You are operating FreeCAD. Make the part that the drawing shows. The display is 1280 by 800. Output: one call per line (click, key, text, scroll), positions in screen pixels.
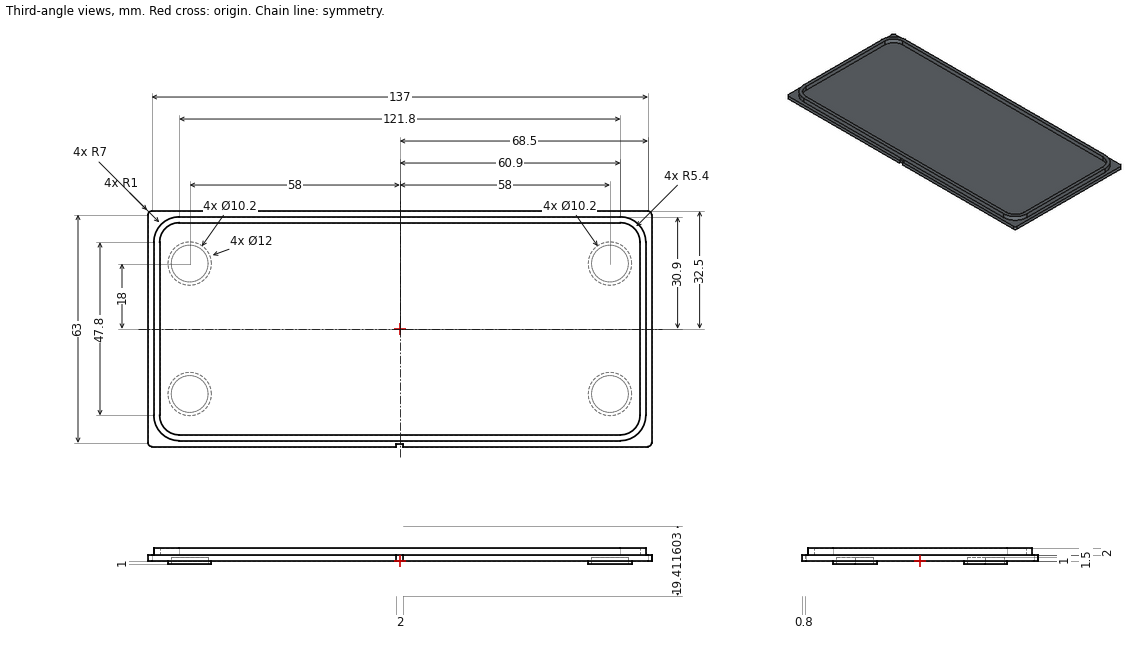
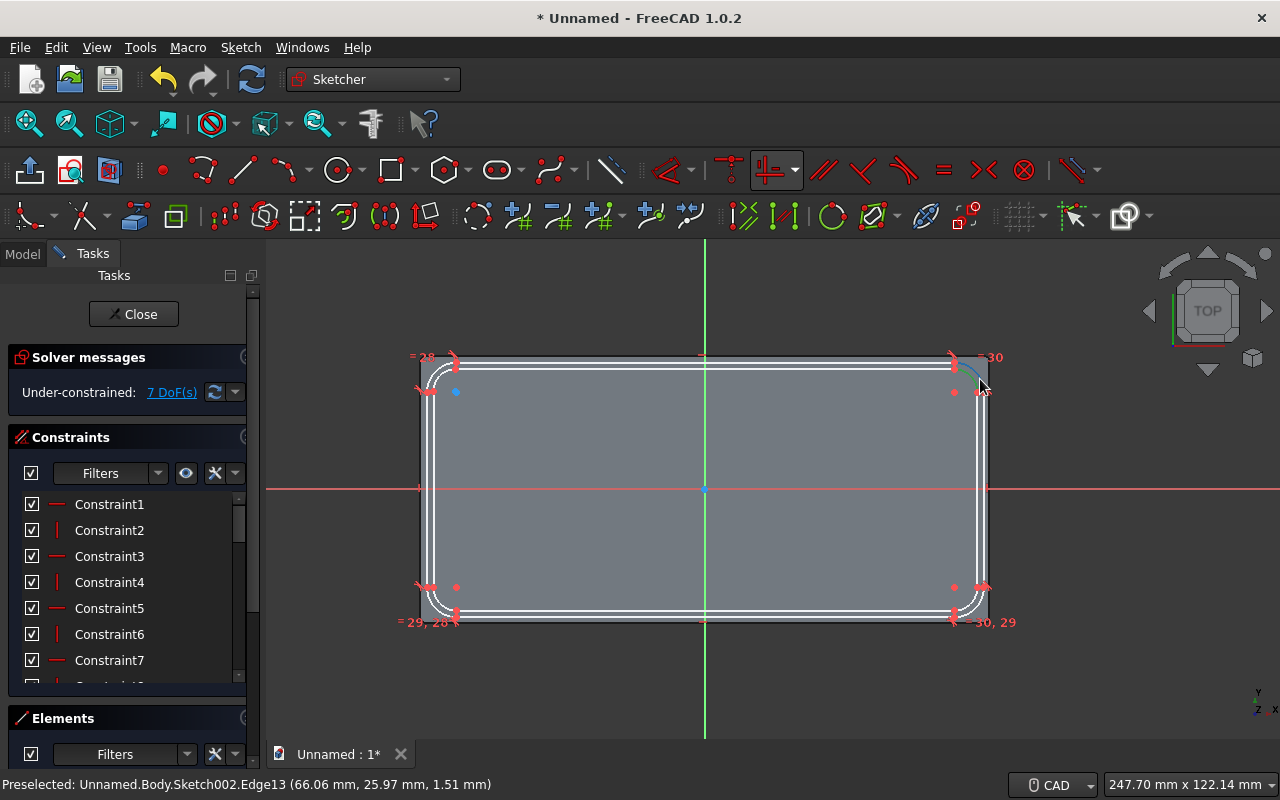
scroll(446, 372, up, 5)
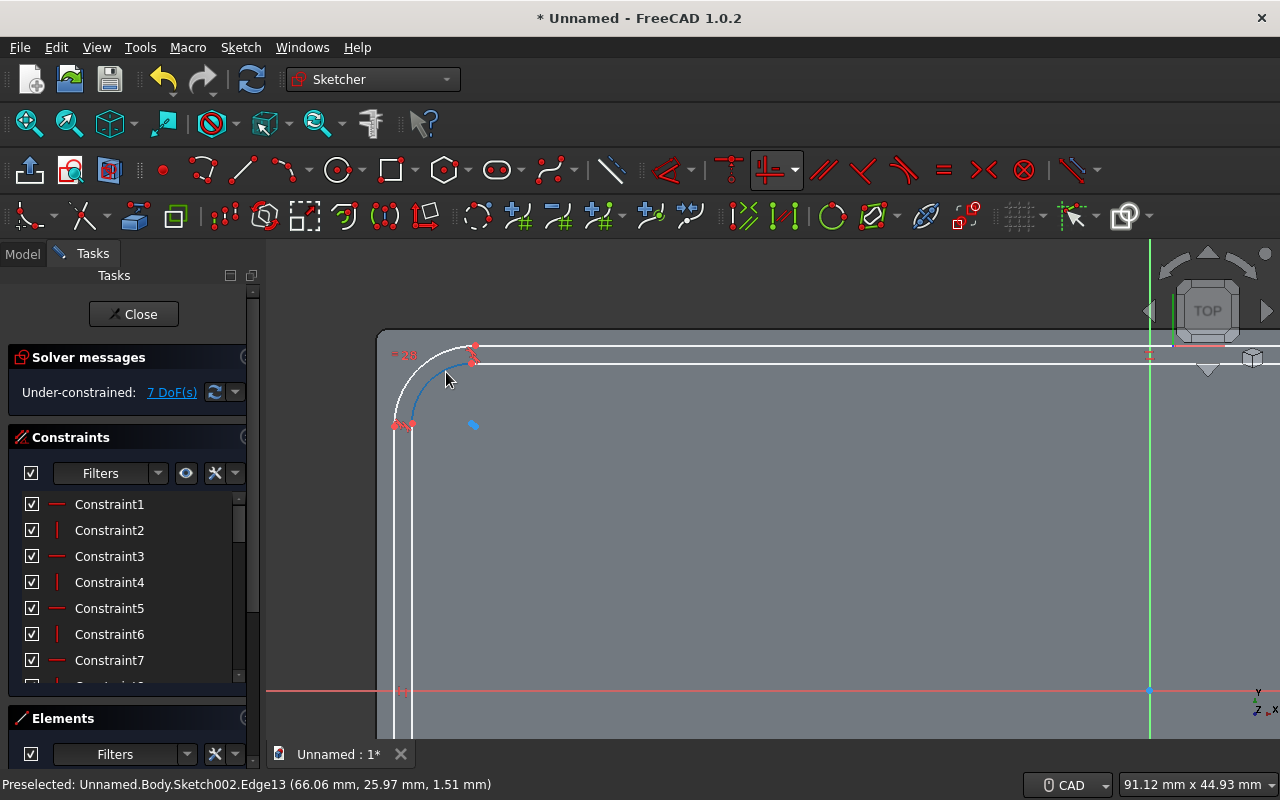
click(445, 370)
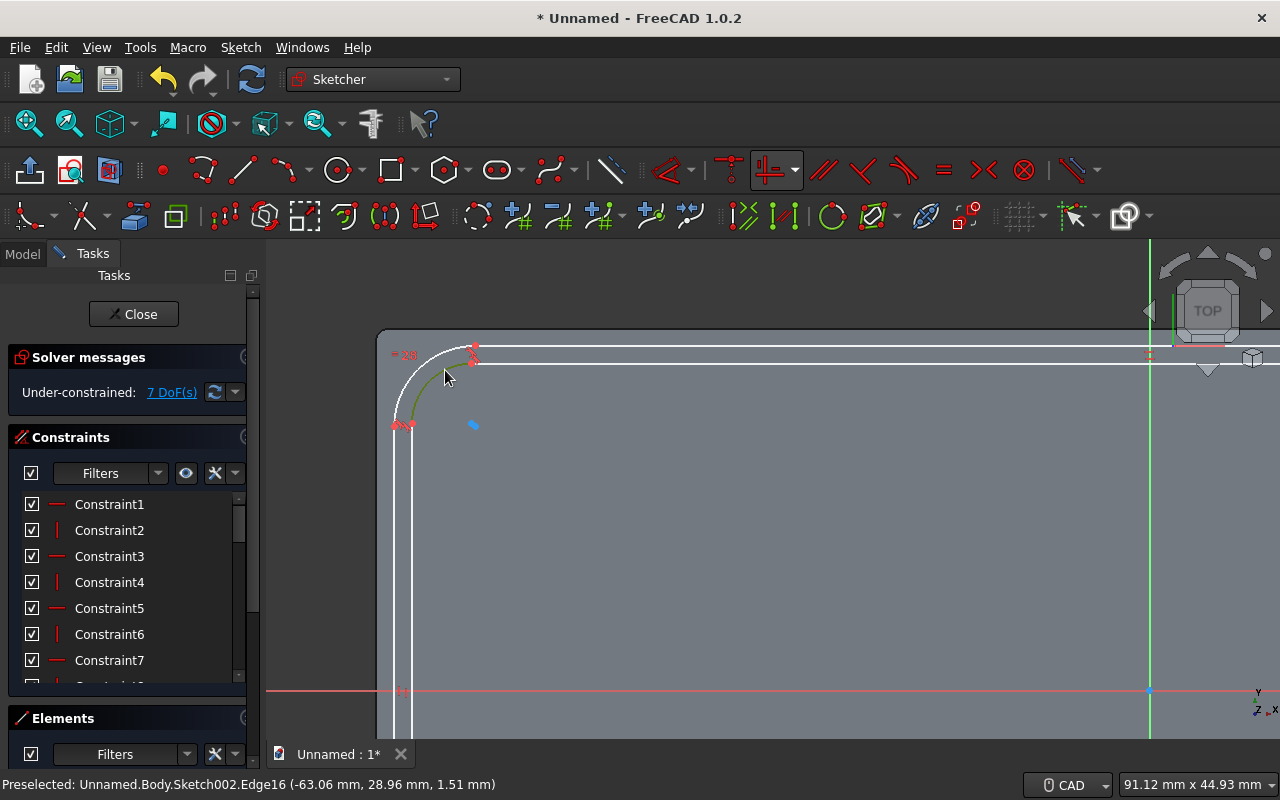
click(944, 170)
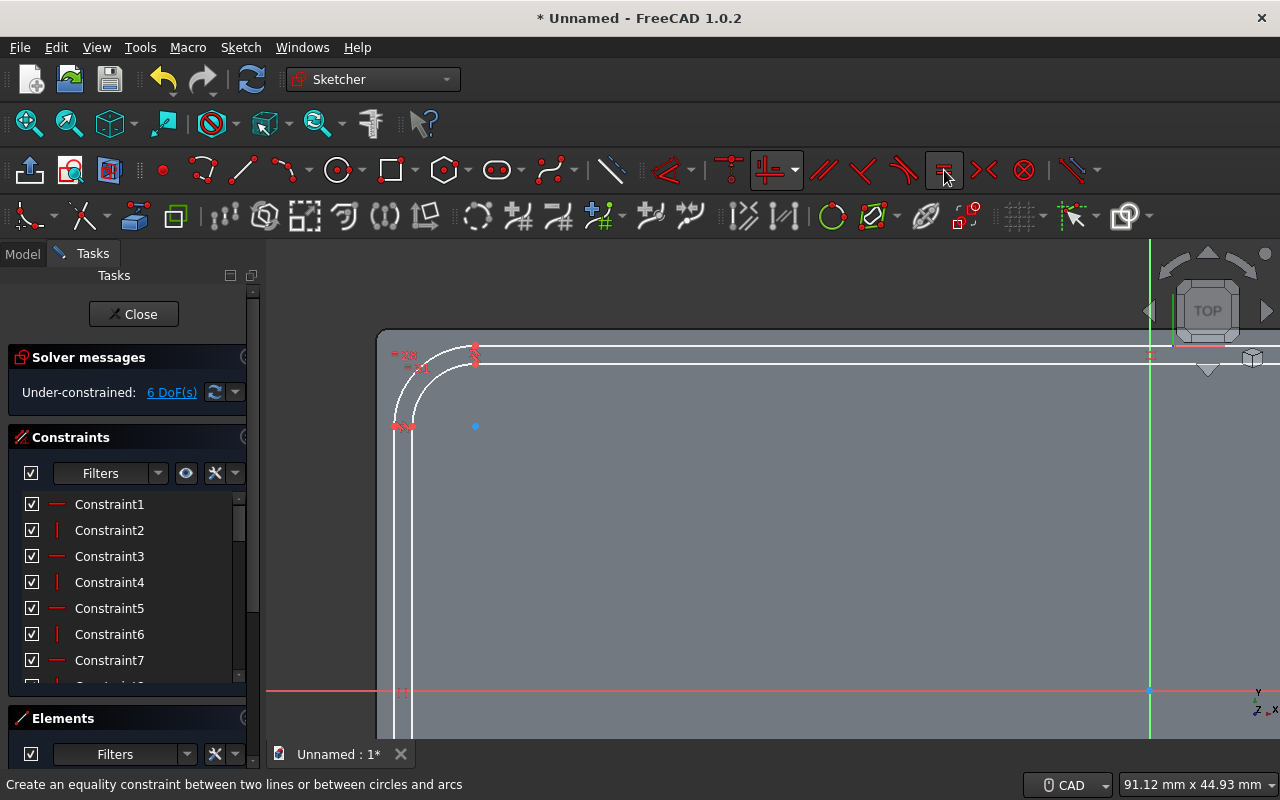
click(666, 170)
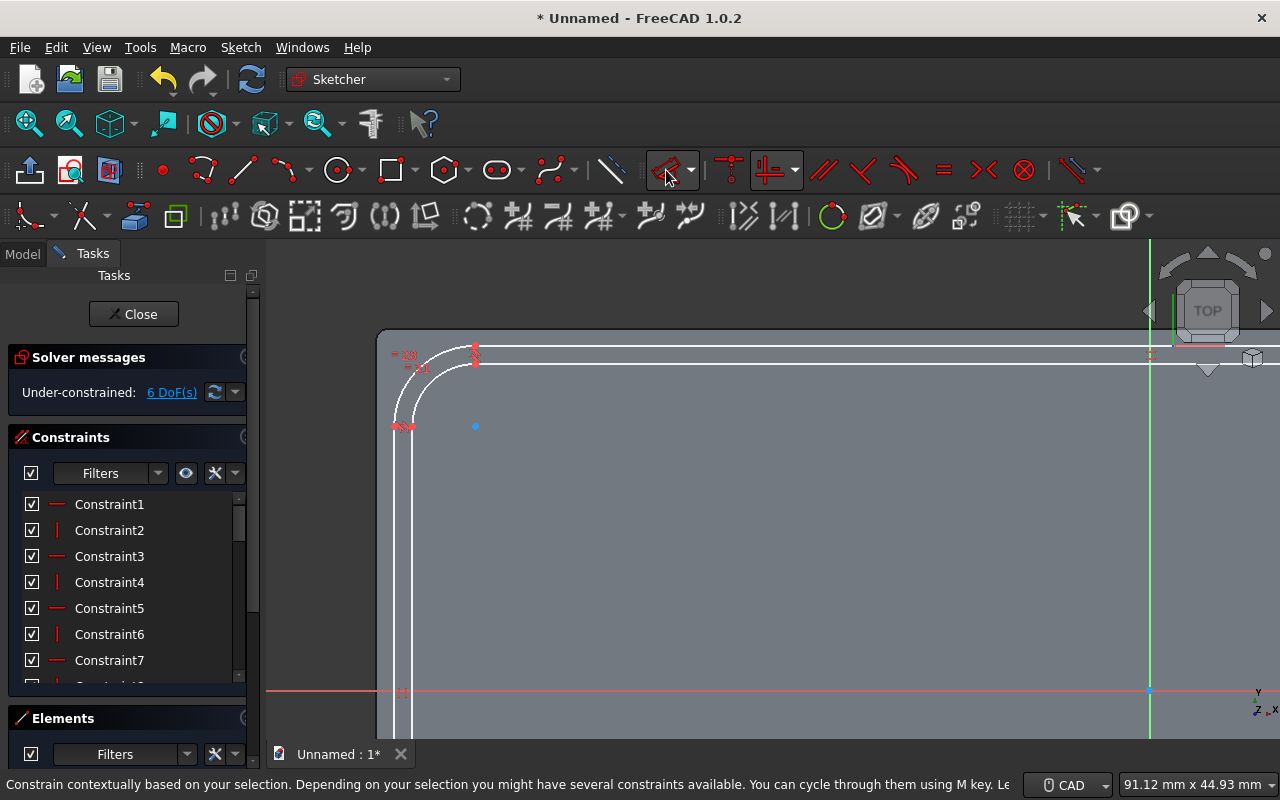
click(438, 355)
click(423, 327)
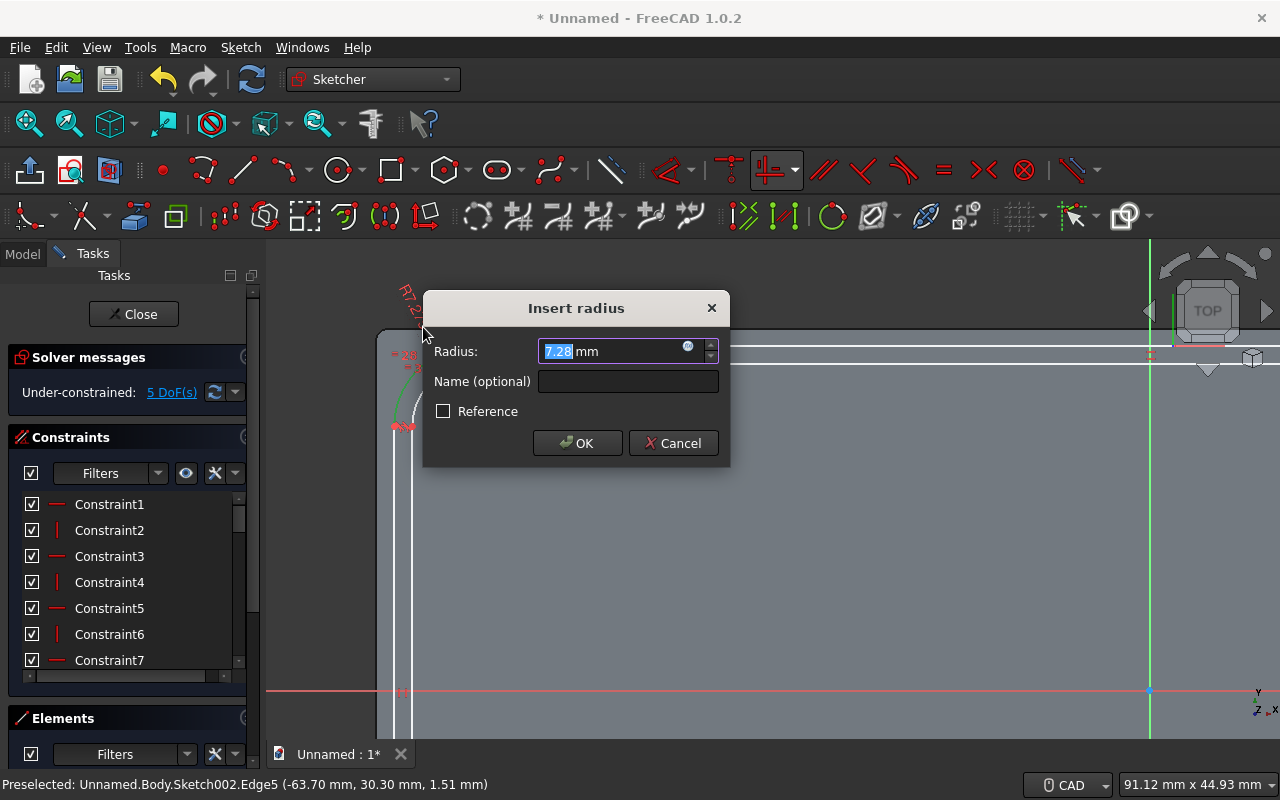
text(7)
key(Return)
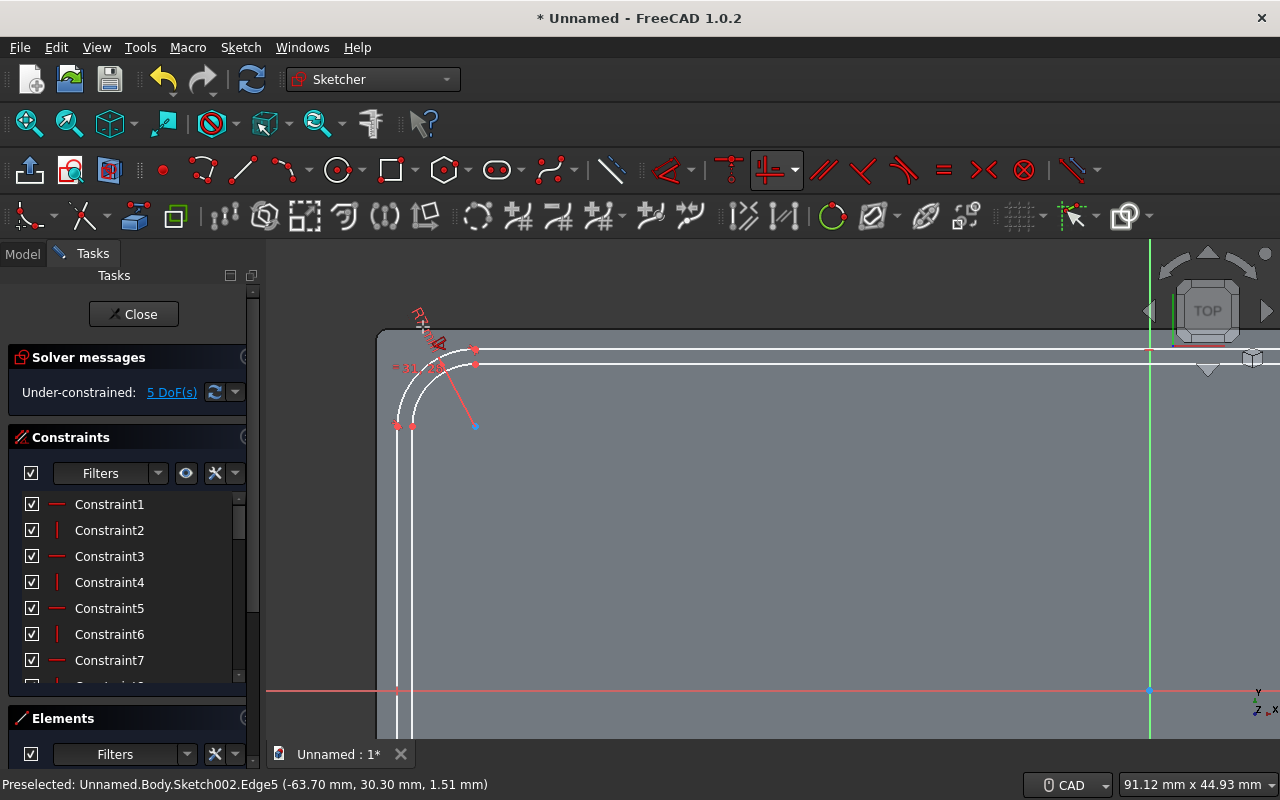
scroll(445, 372, down, 5)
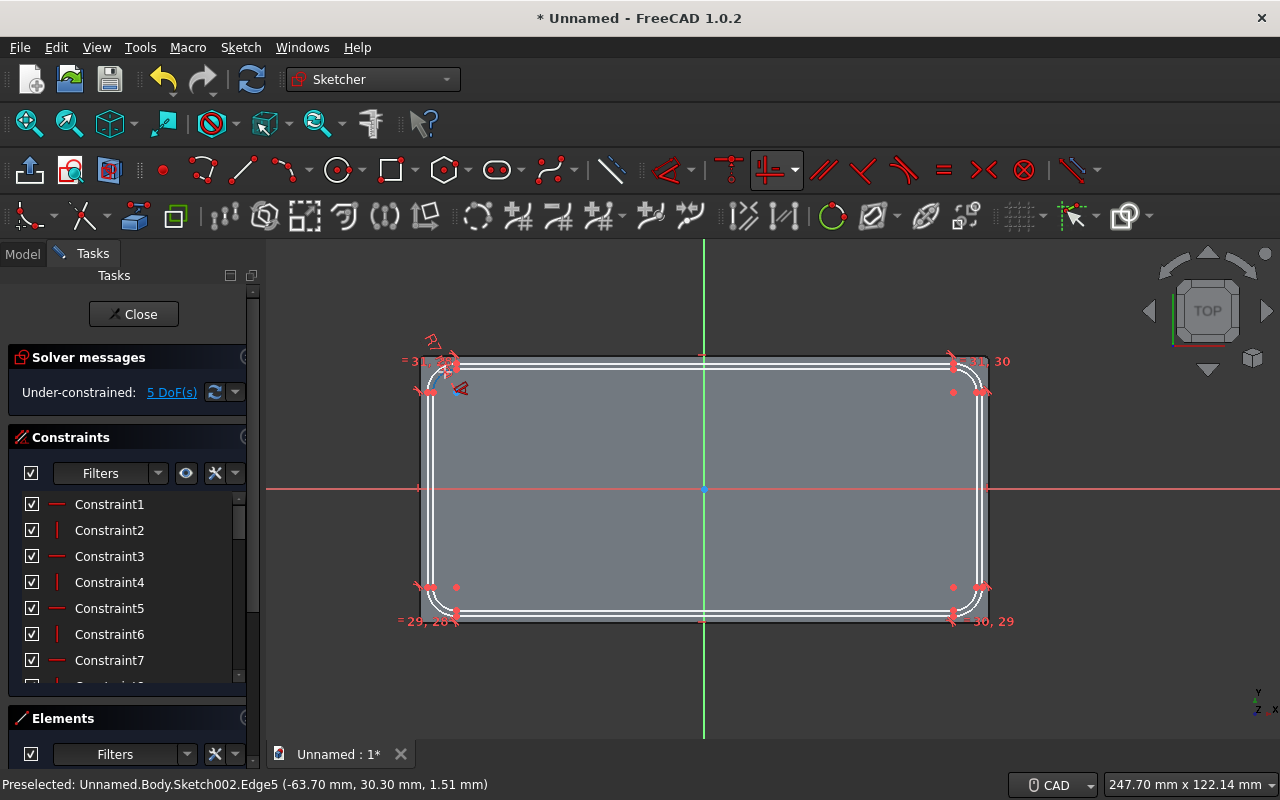
scroll(974, 382, up, 5)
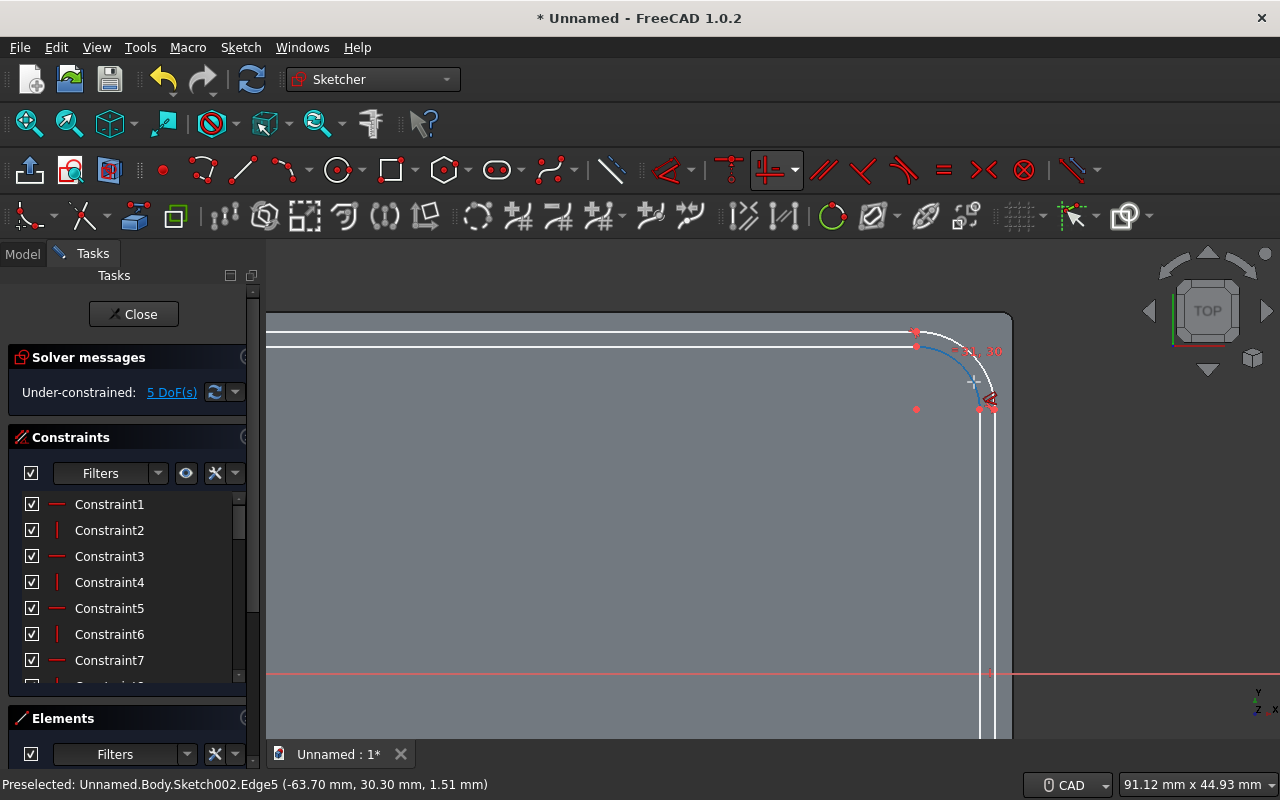
click(973, 381)
click(1001, 366)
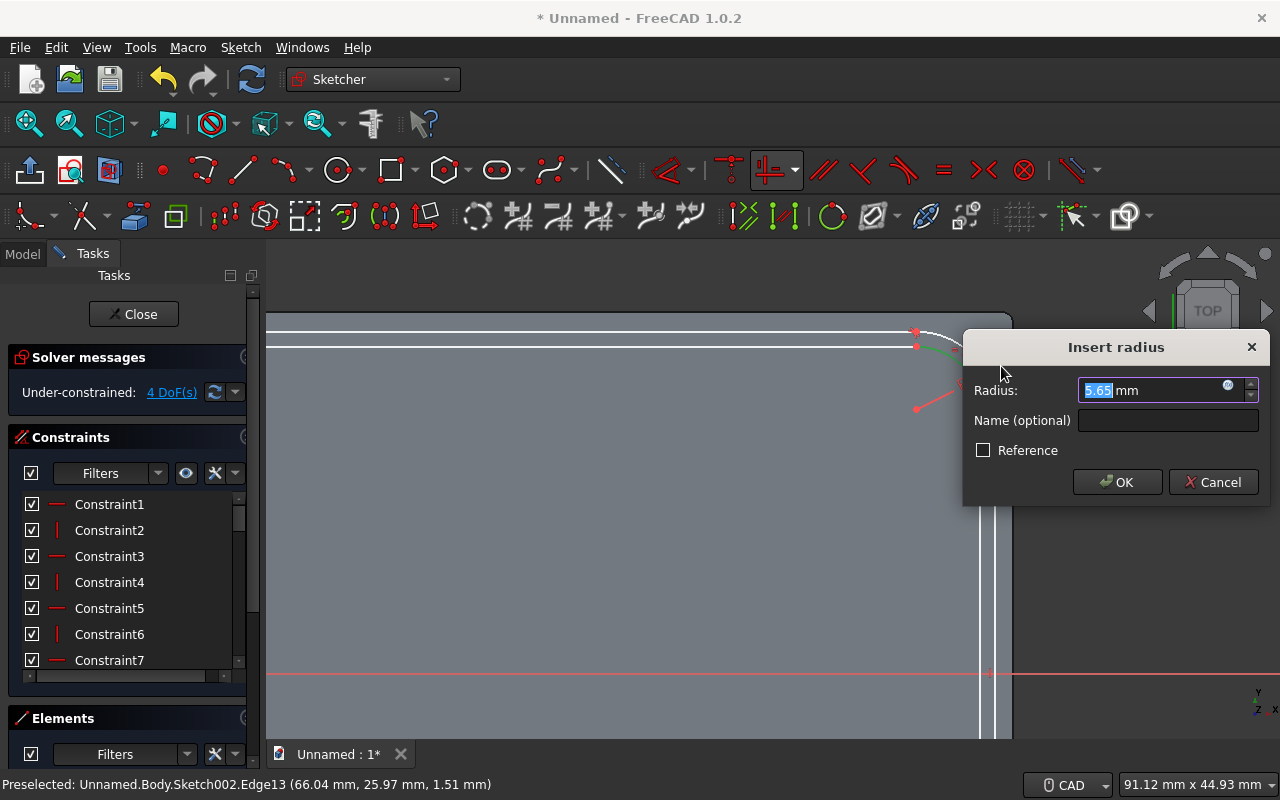
text(5.4)
key(Return)